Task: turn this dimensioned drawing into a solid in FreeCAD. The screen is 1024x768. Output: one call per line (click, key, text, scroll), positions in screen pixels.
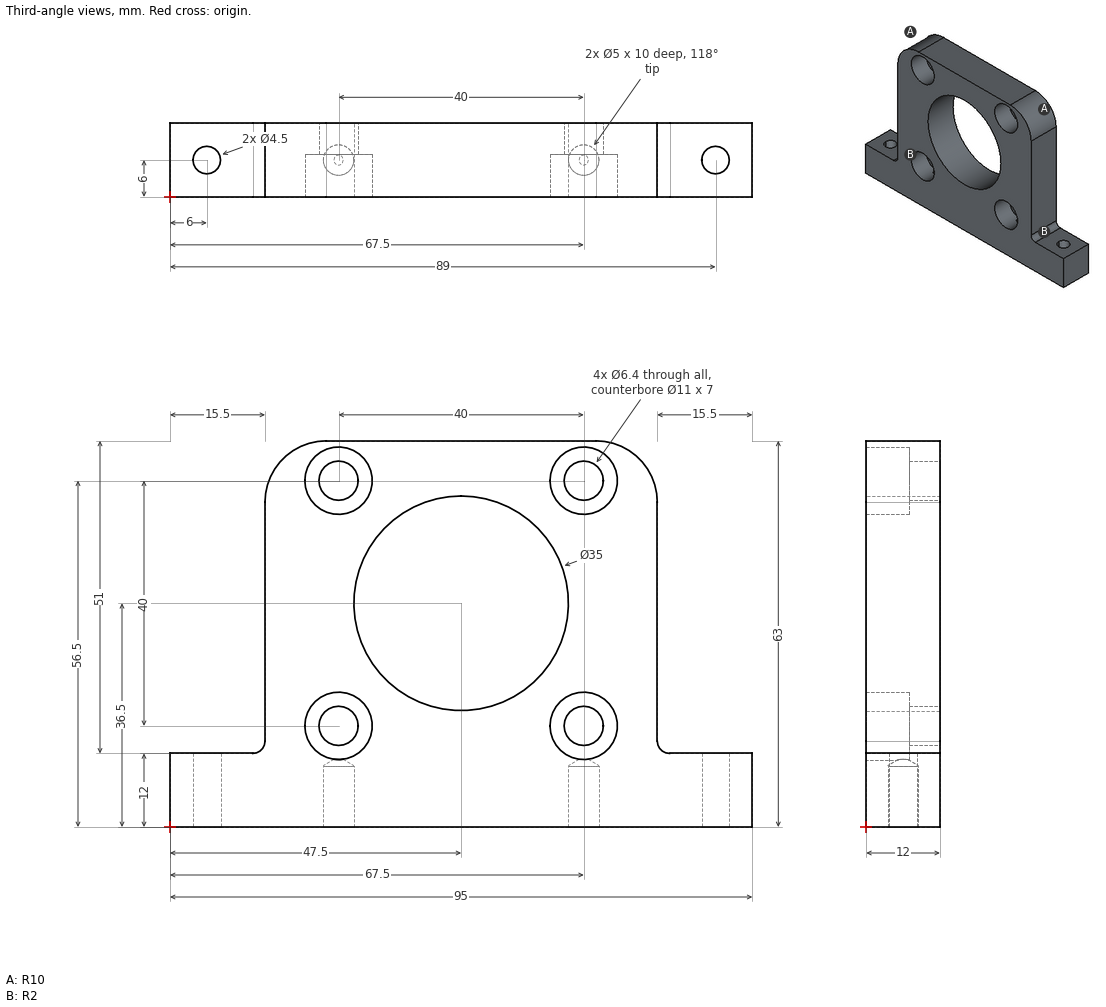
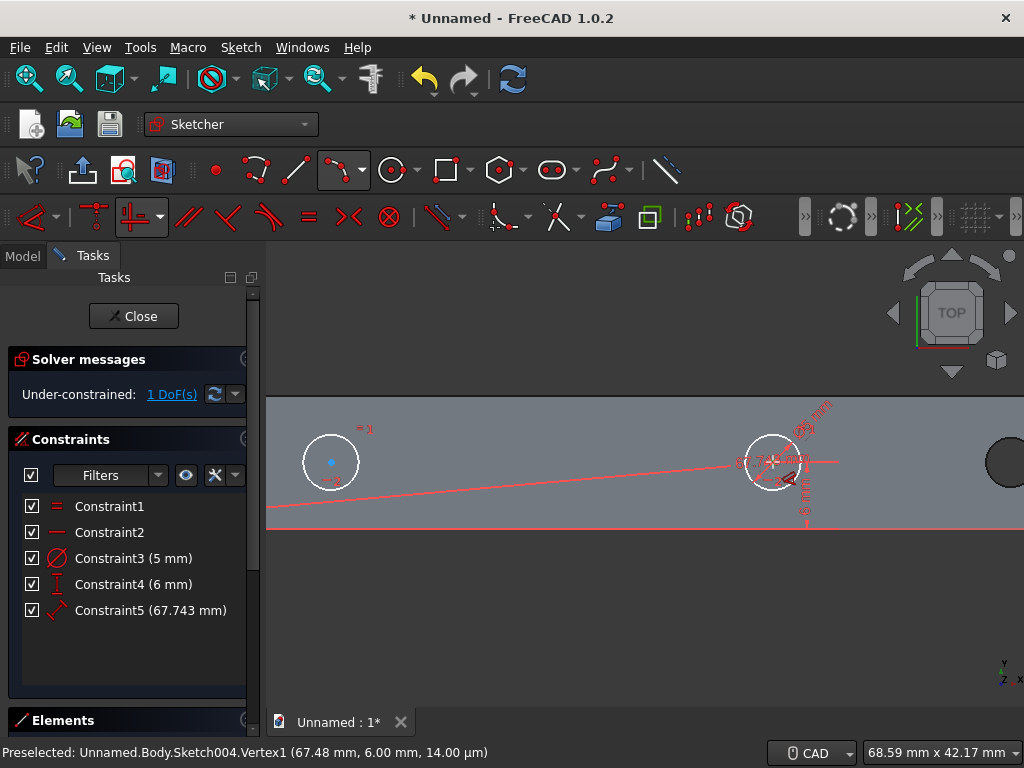
click(331, 462)
click(552, 428)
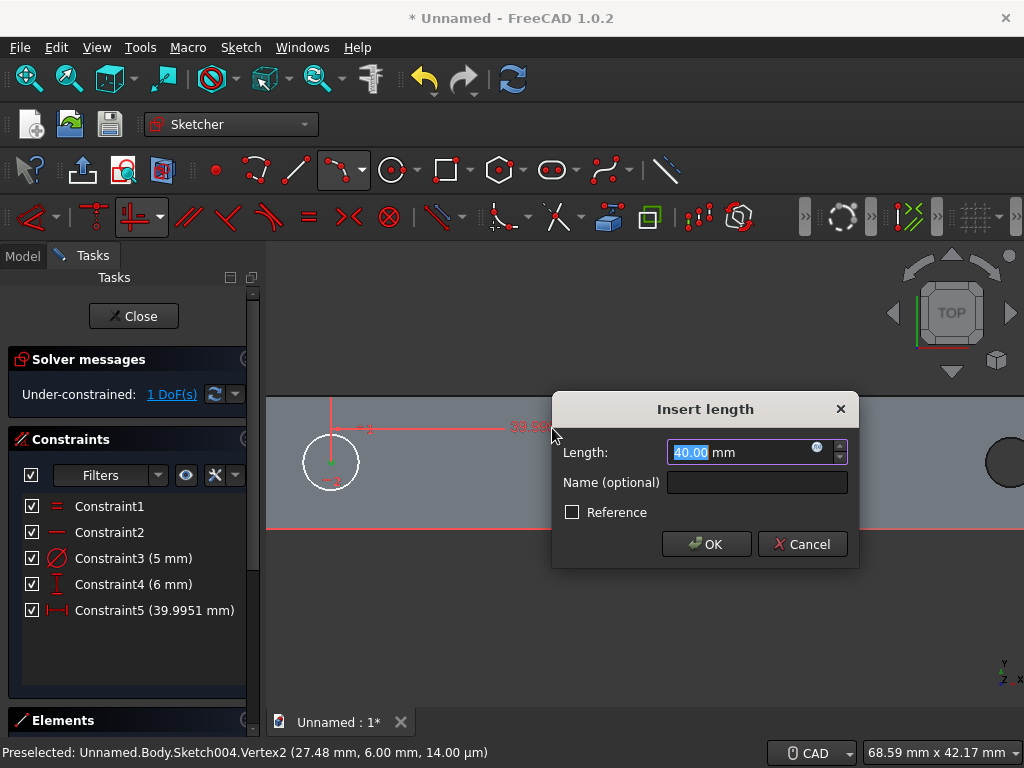
text(40)
key(Return)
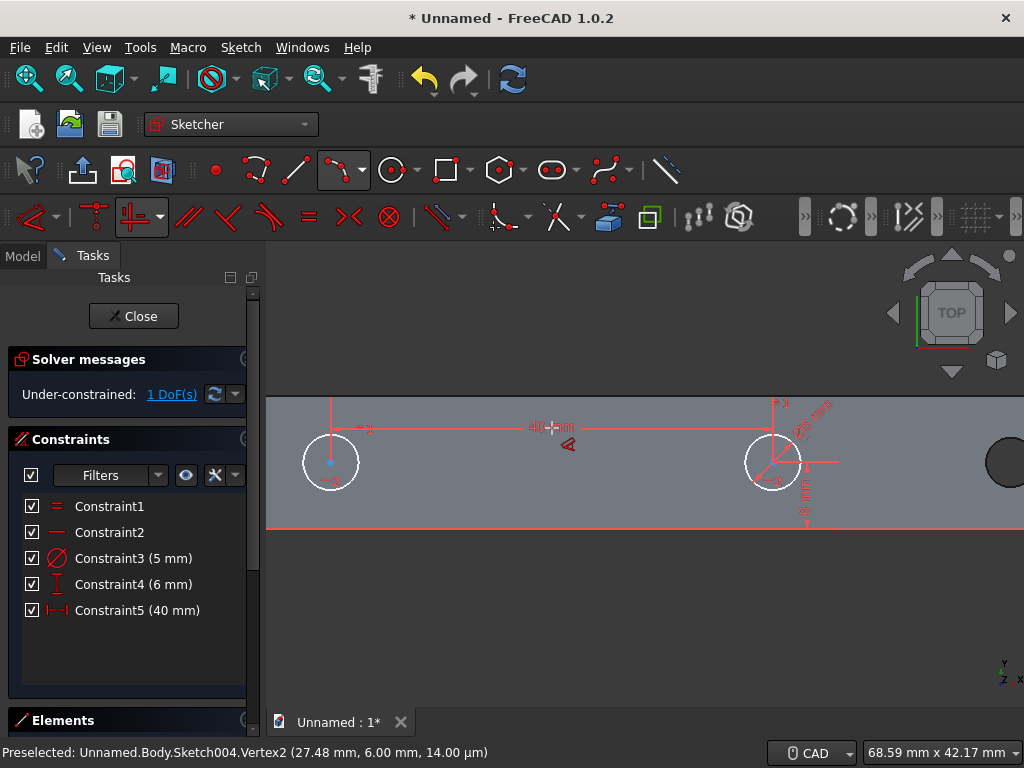
click(773, 462)
click(533, 563)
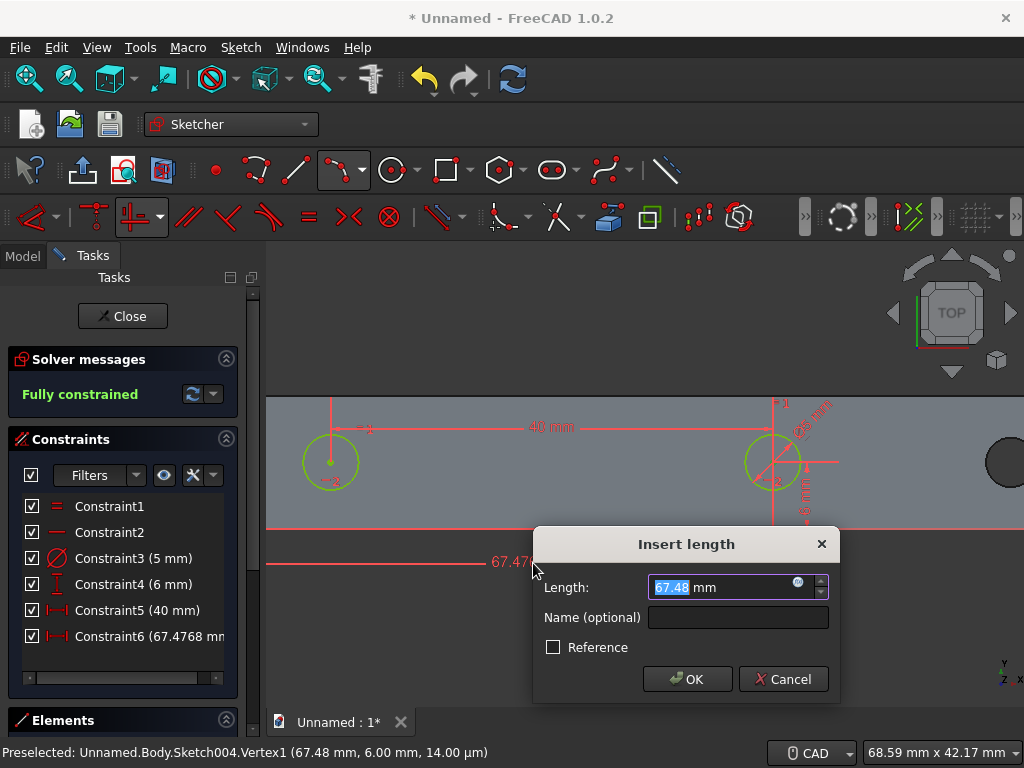
text(67.5)
key(Return)
key(Escape)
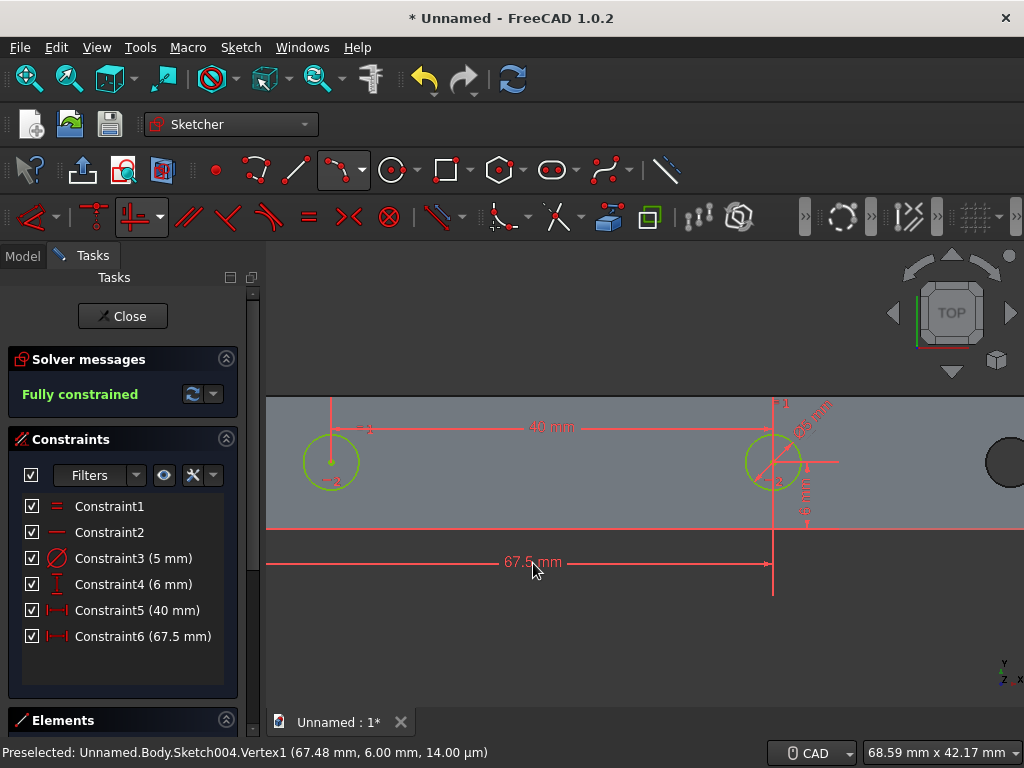
click(123, 316)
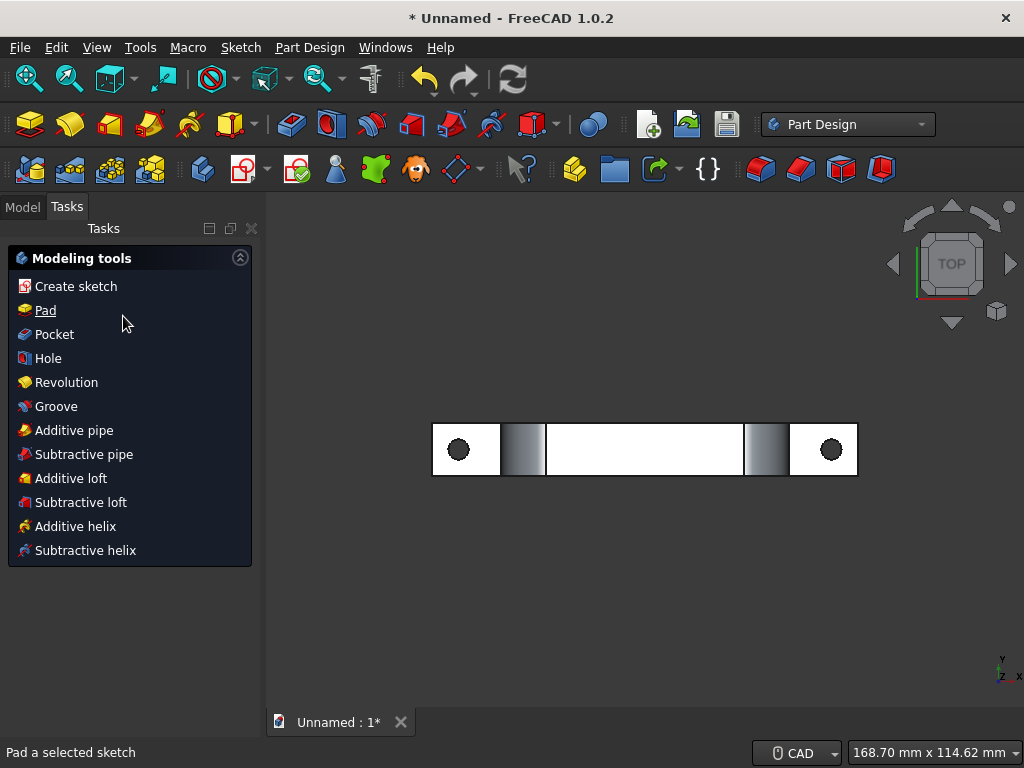
click(332, 124)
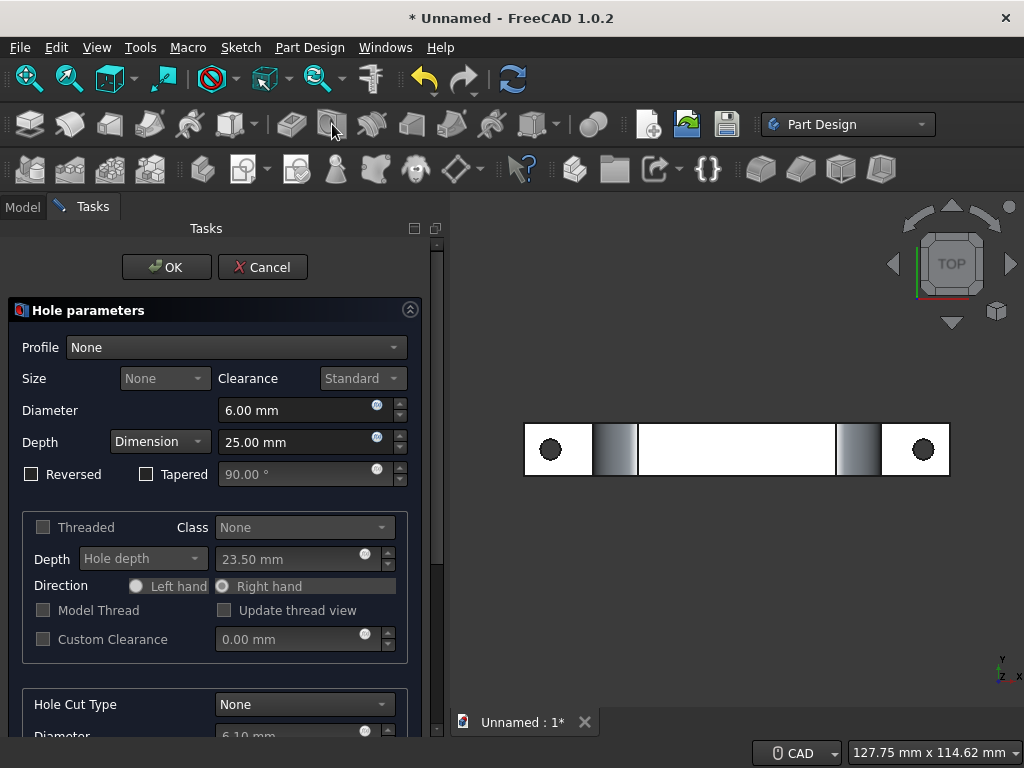
triple_click(305, 410)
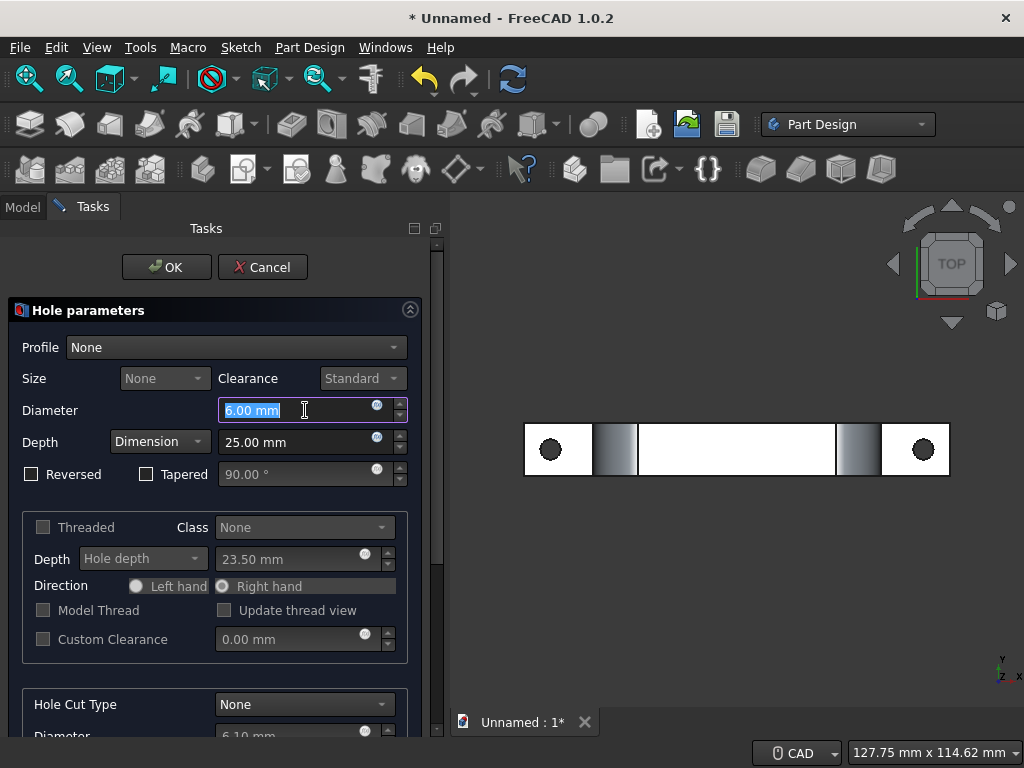
text(5)
key(Tab)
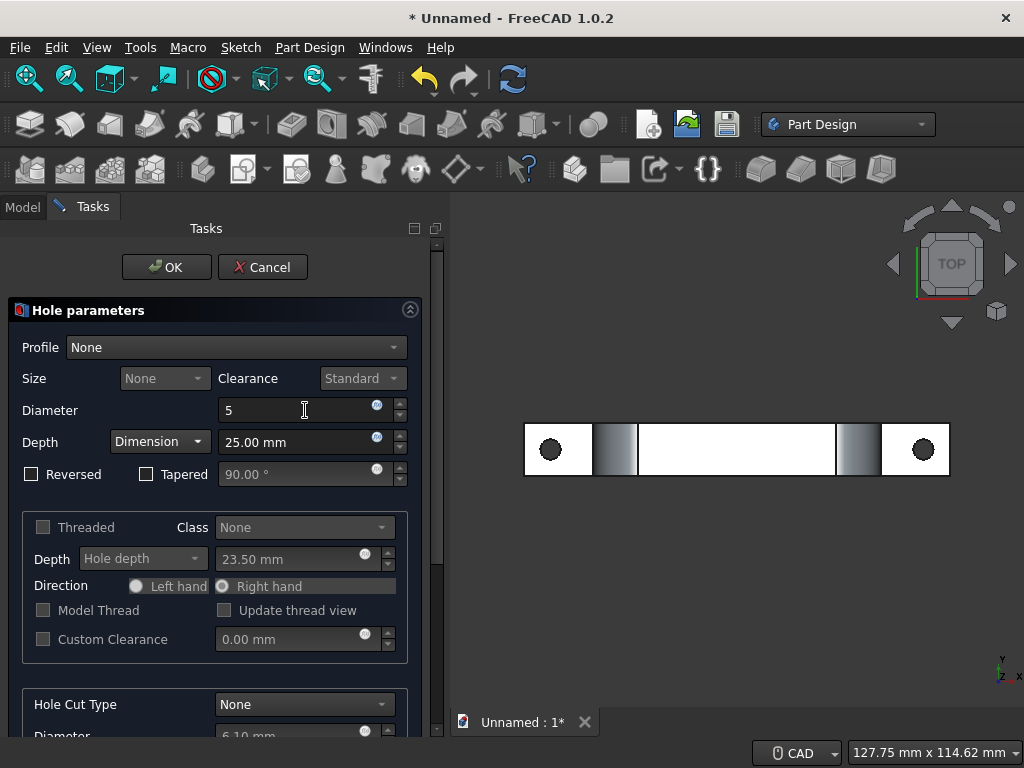
triple_click(305, 442)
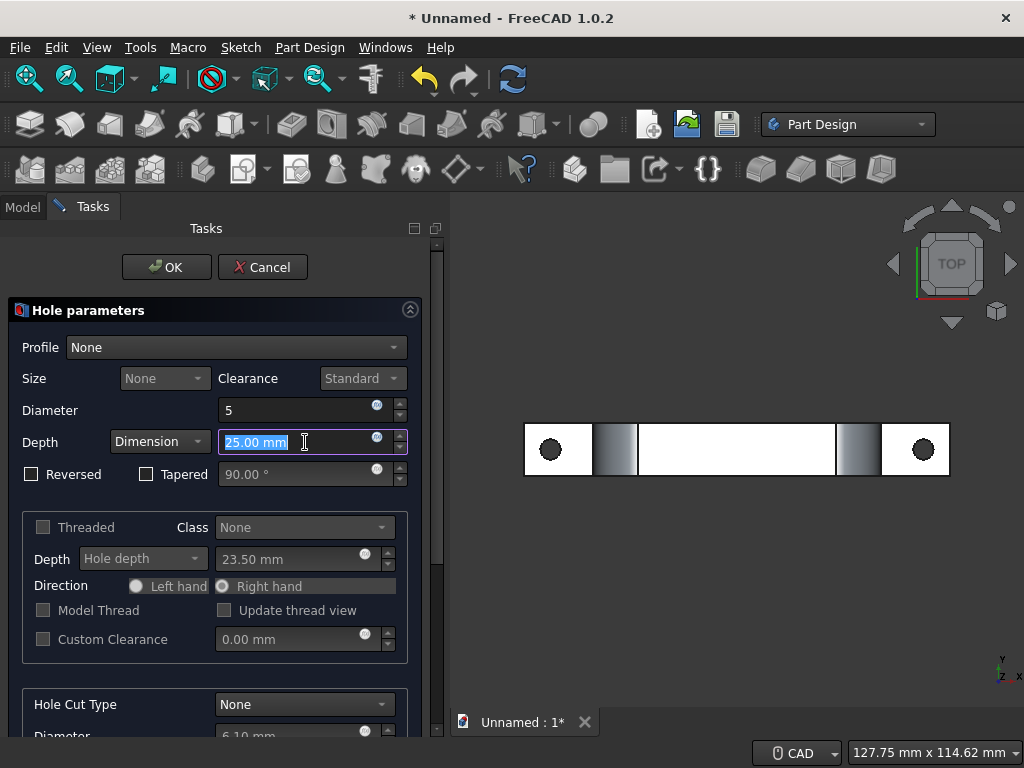
text(10)
key(Tab)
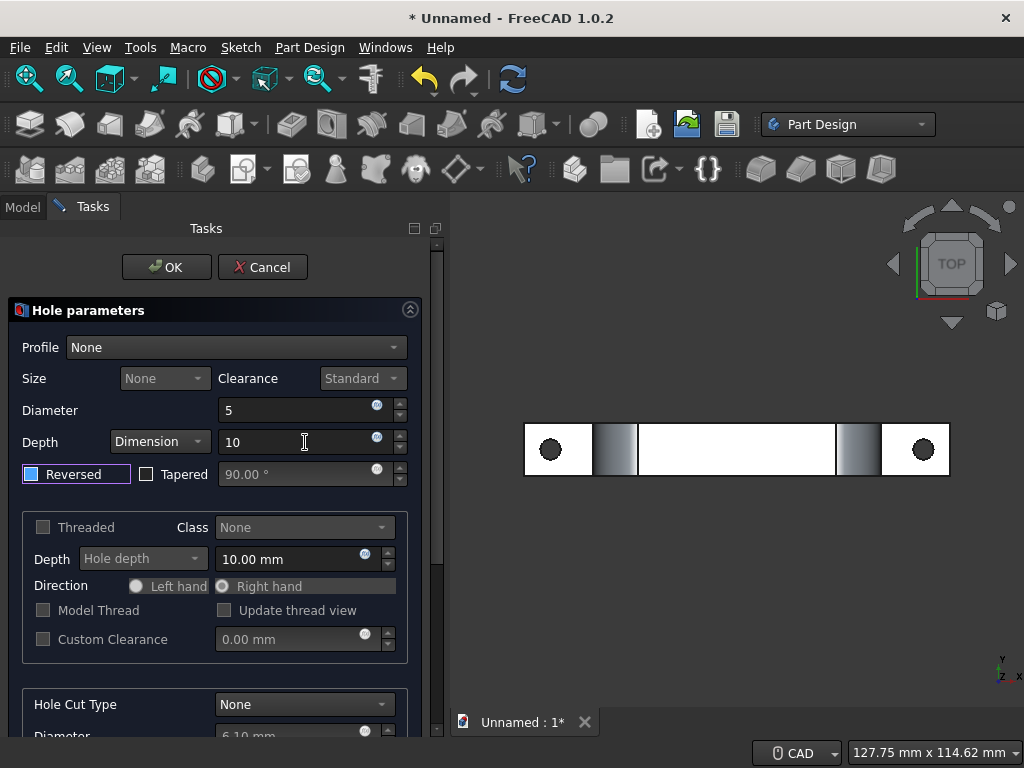
click(30, 474)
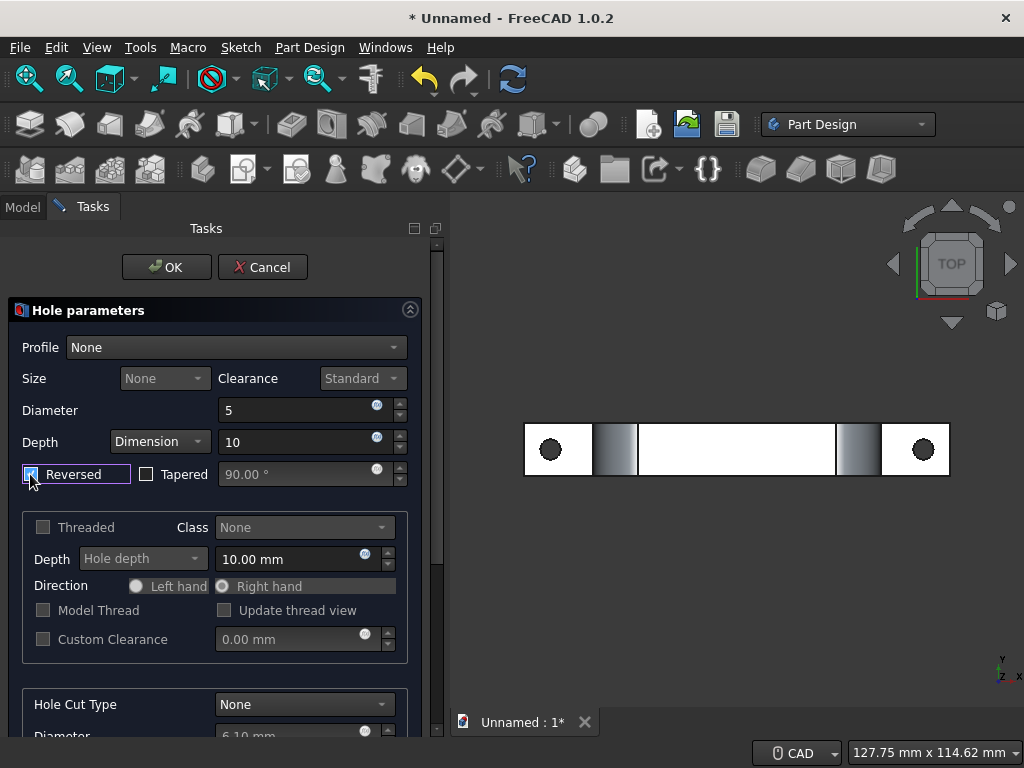
click(167, 267)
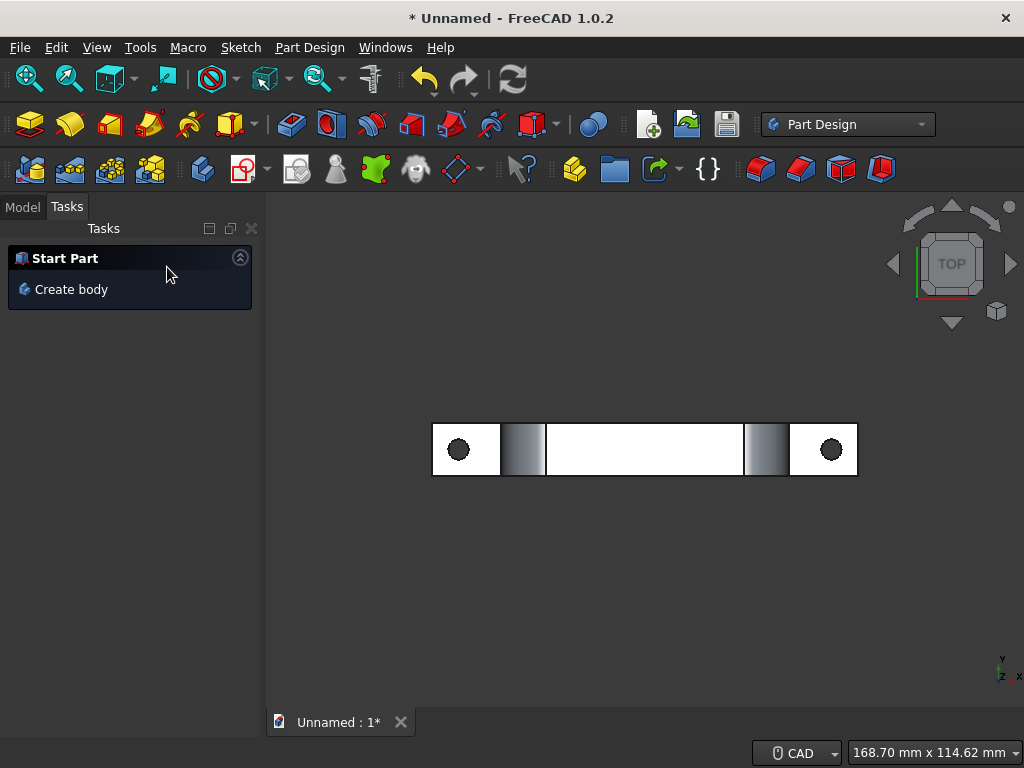
key(0)